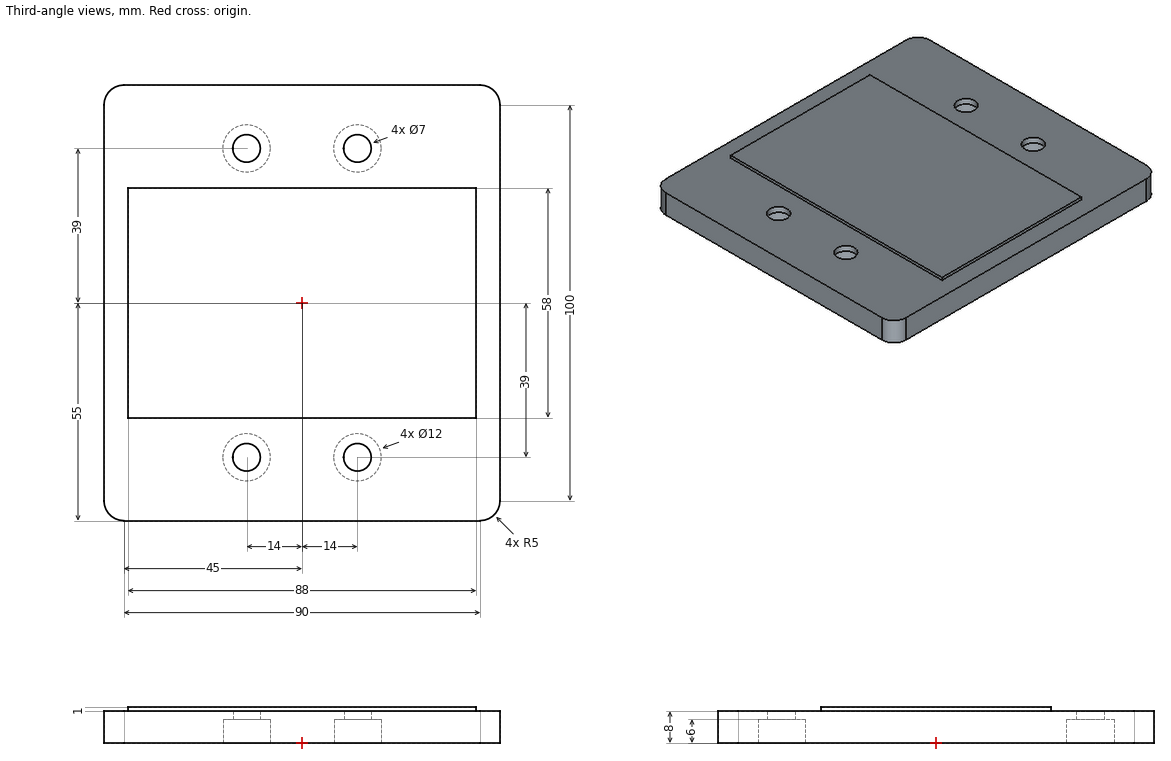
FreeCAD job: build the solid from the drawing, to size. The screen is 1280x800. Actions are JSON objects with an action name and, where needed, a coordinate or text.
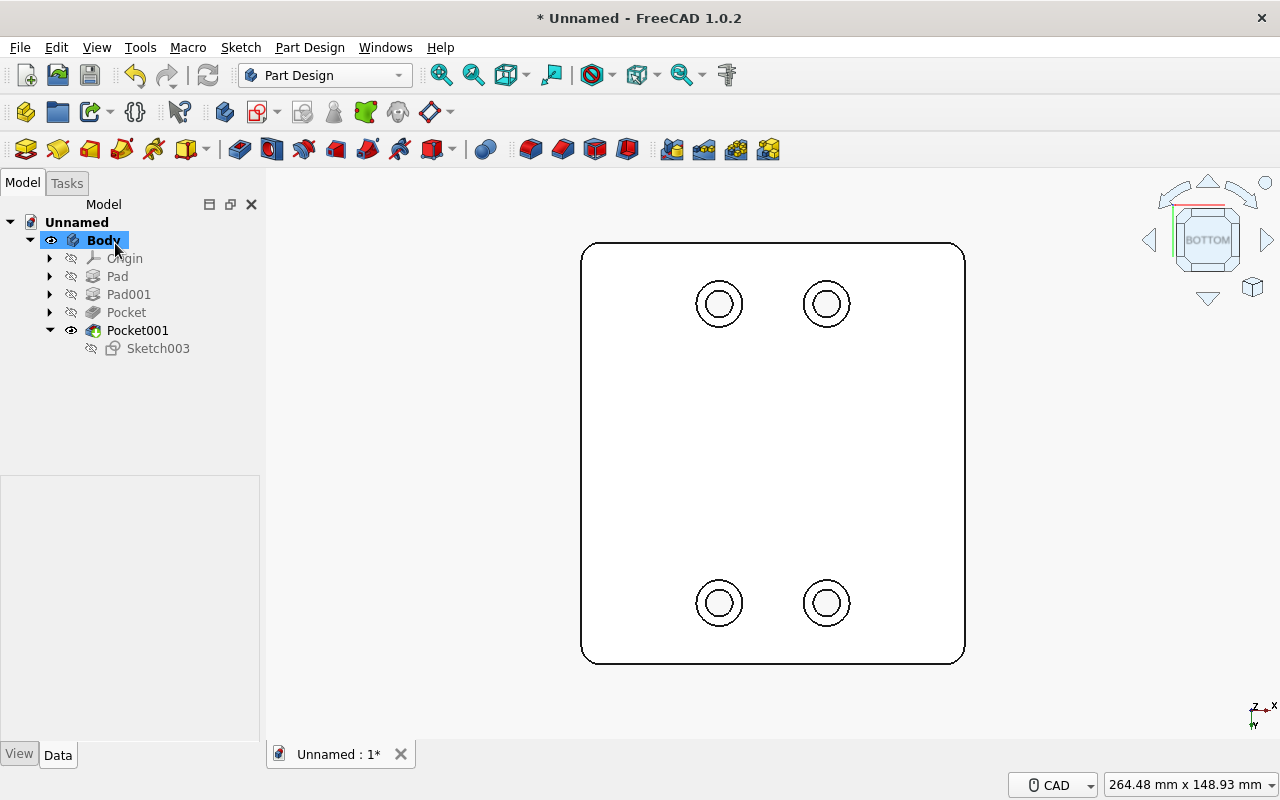
{"action": "key", "text": "0"}